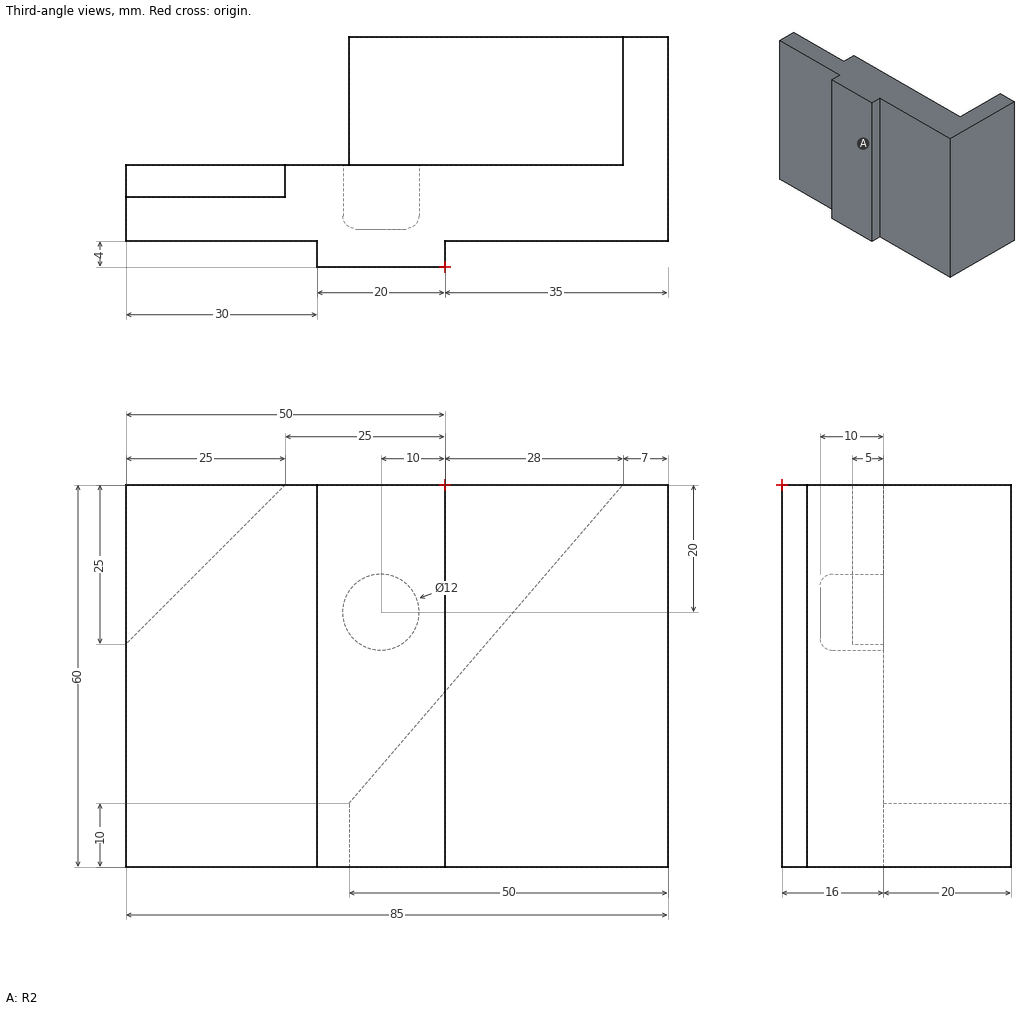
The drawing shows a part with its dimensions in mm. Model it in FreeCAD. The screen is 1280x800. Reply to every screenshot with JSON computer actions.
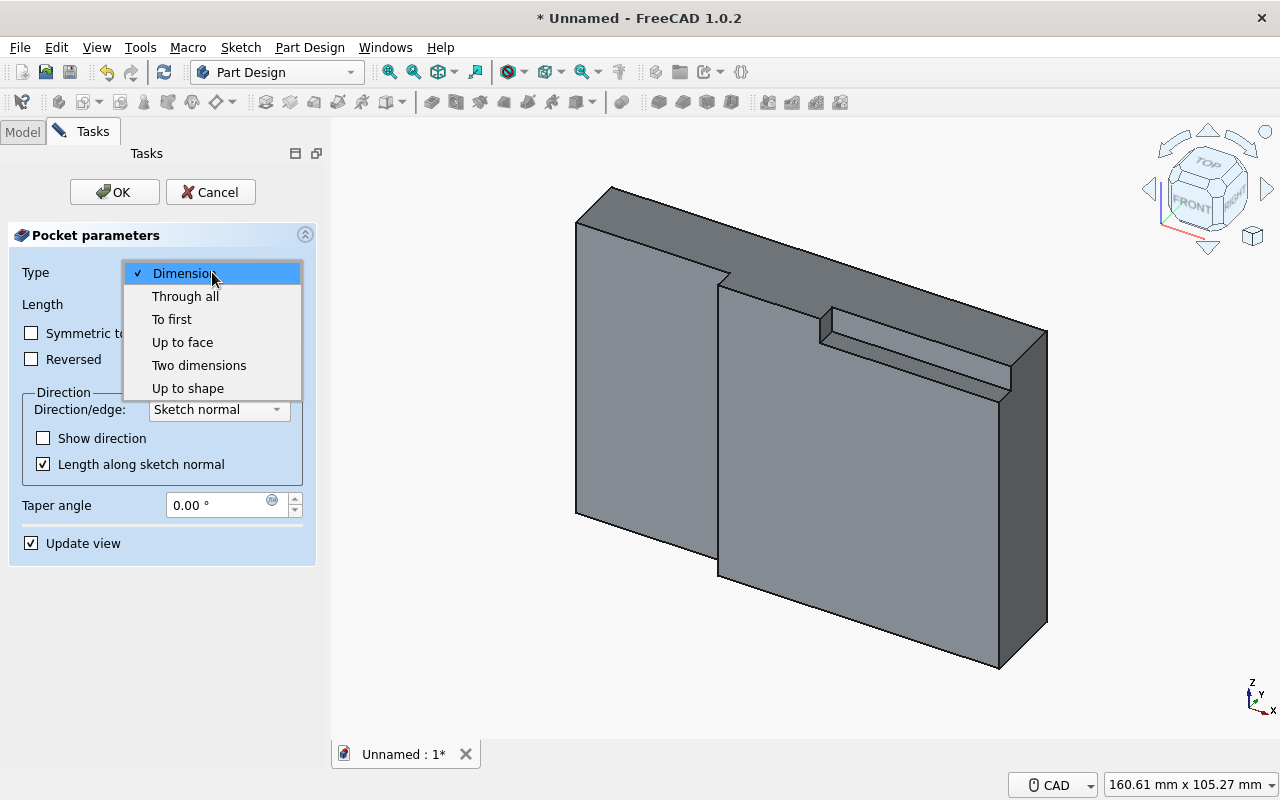
{"action": "left_click", "coordinate": [212, 296]}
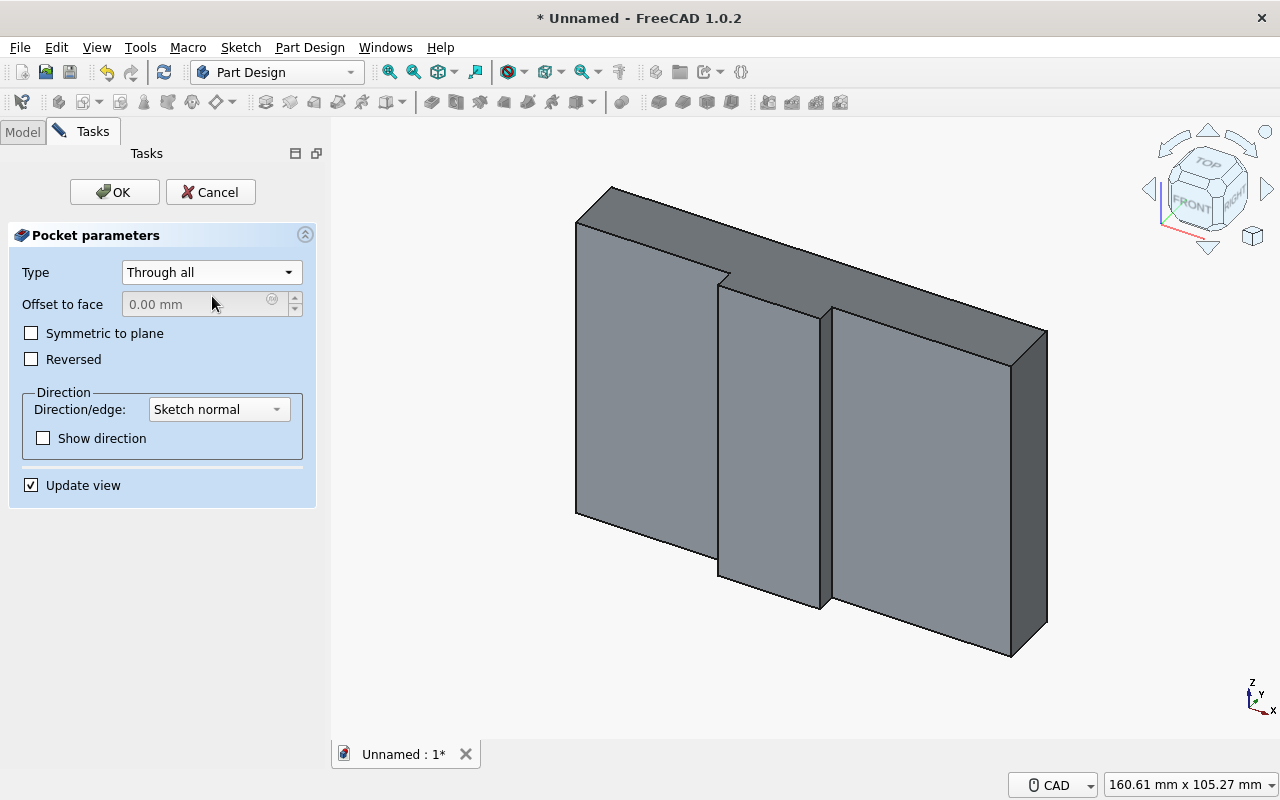
{"action": "left_click", "coordinate": [115, 192]}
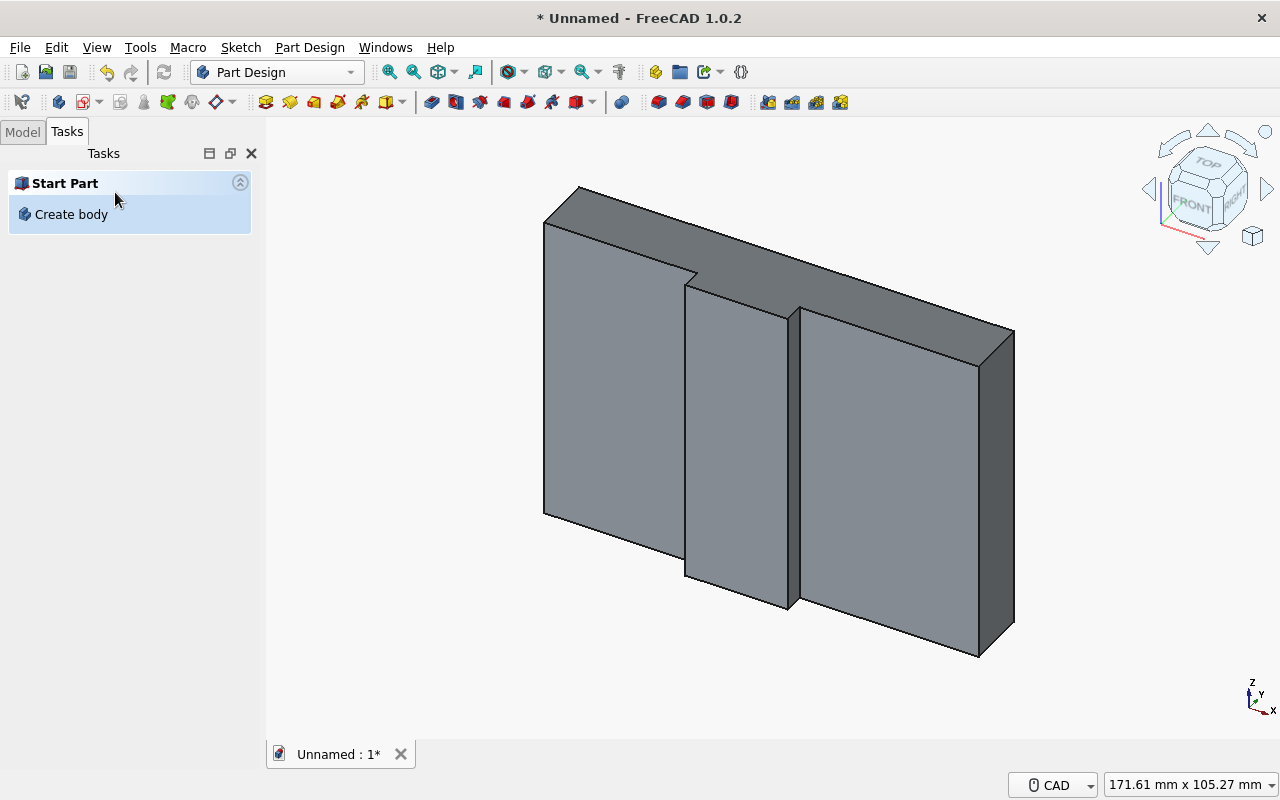
{"action": "key", "text": "4"}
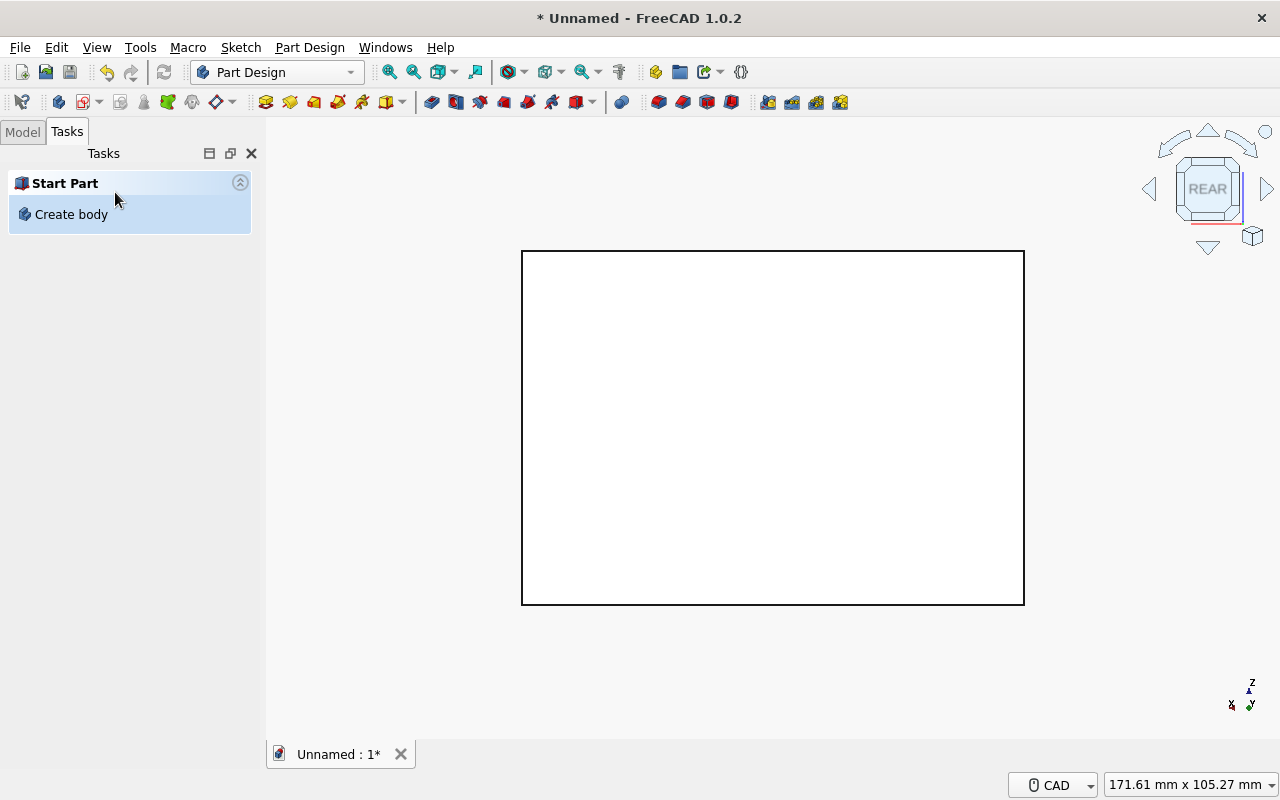
{"action": "left_click", "coordinate": [701, 427]}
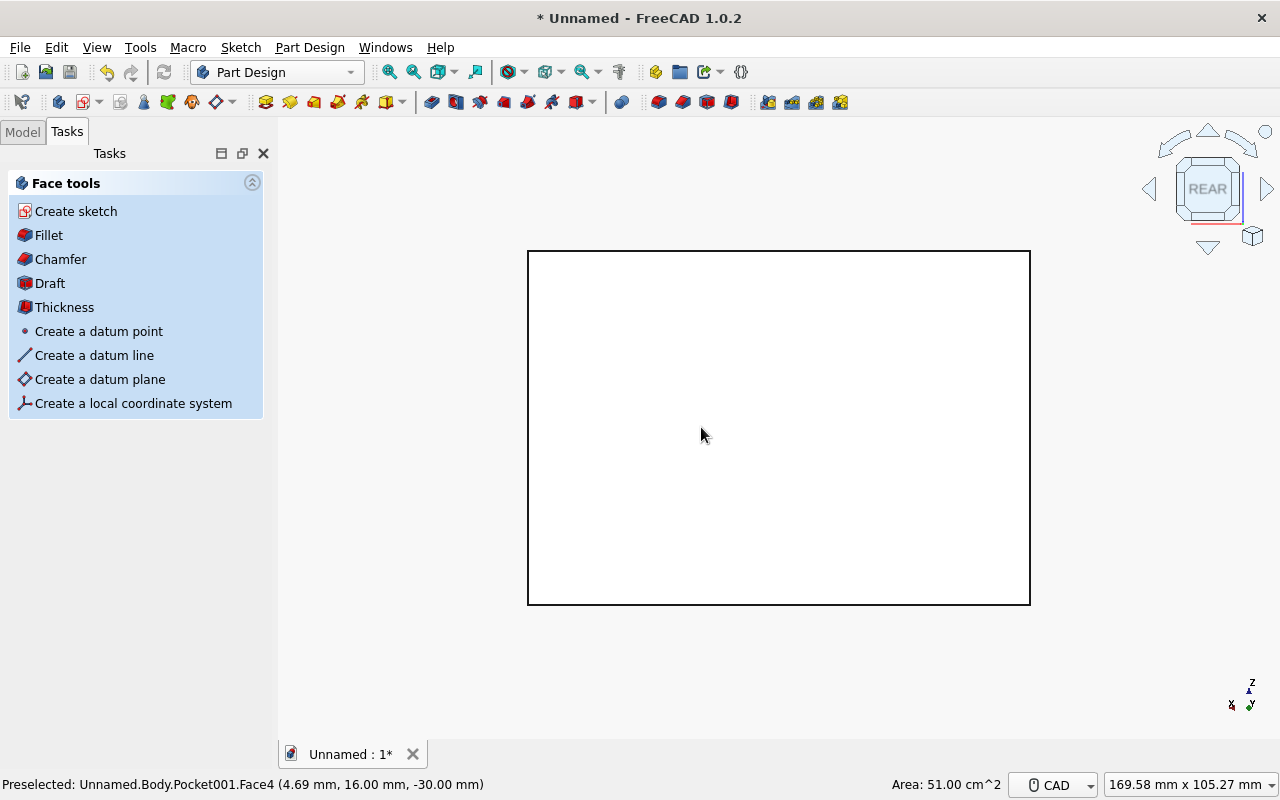
{"action": "left_click", "coordinate": [84, 102]}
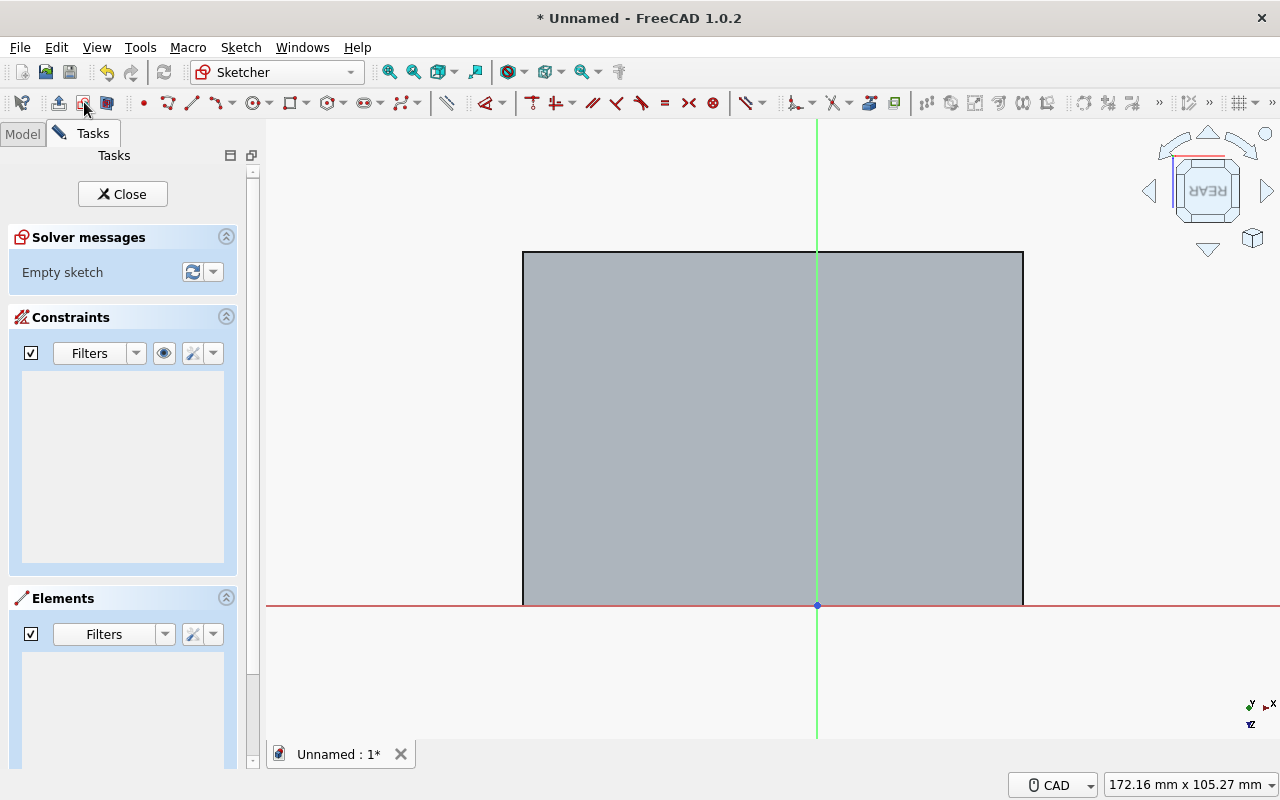
{"action": "left_click", "coordinate": [168, 104]}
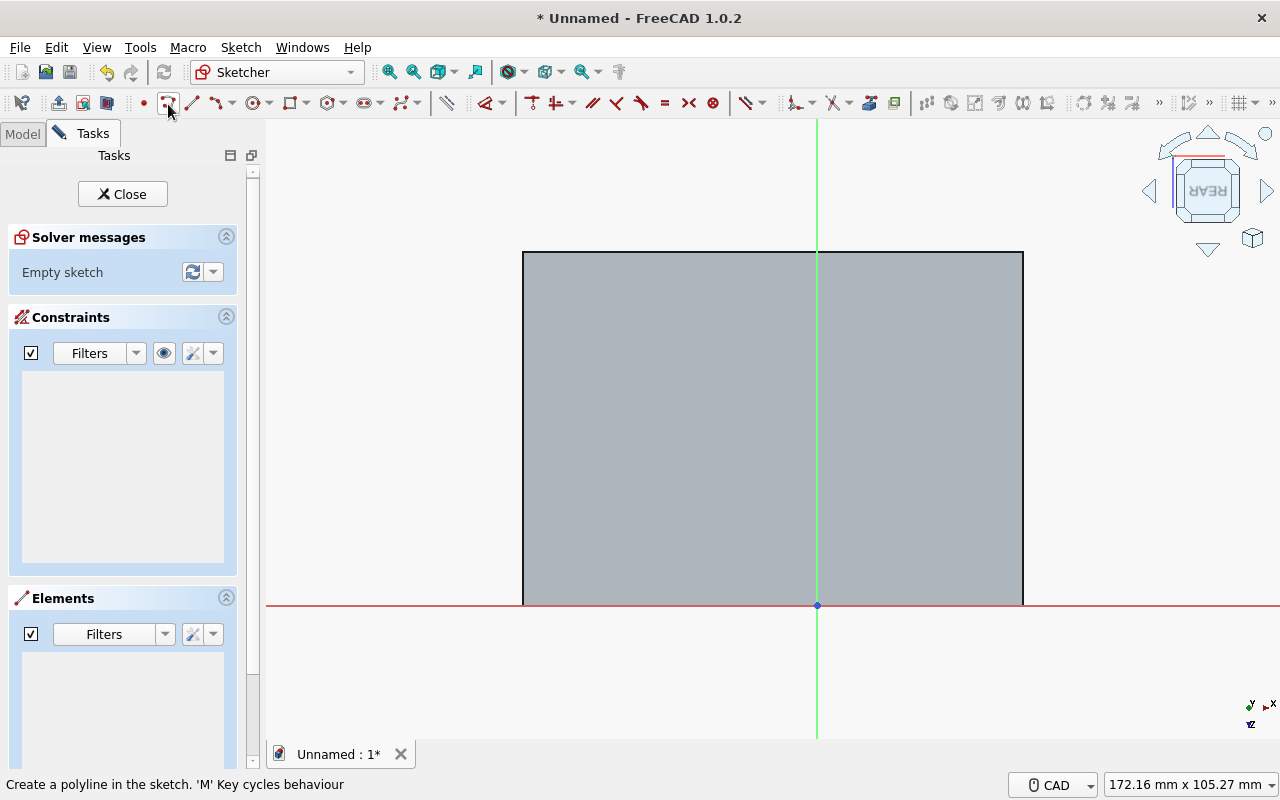
{"action": "left_click", "coordinate": [982, 606]}
{"action": "left_click", "coordinate": [1023, 597]}
{"action": "left_click", "coordinate": [1023, 252]}
{"action": "left_click", "coordinate": [729, 252]}
{"action": "left_click", "coordinate": [729, 311]}
{"action": "left_click", "coordinate": [982, 606]}
{"action": "key", "text": "Escape"}
{"action": "key", "text": "Escape"}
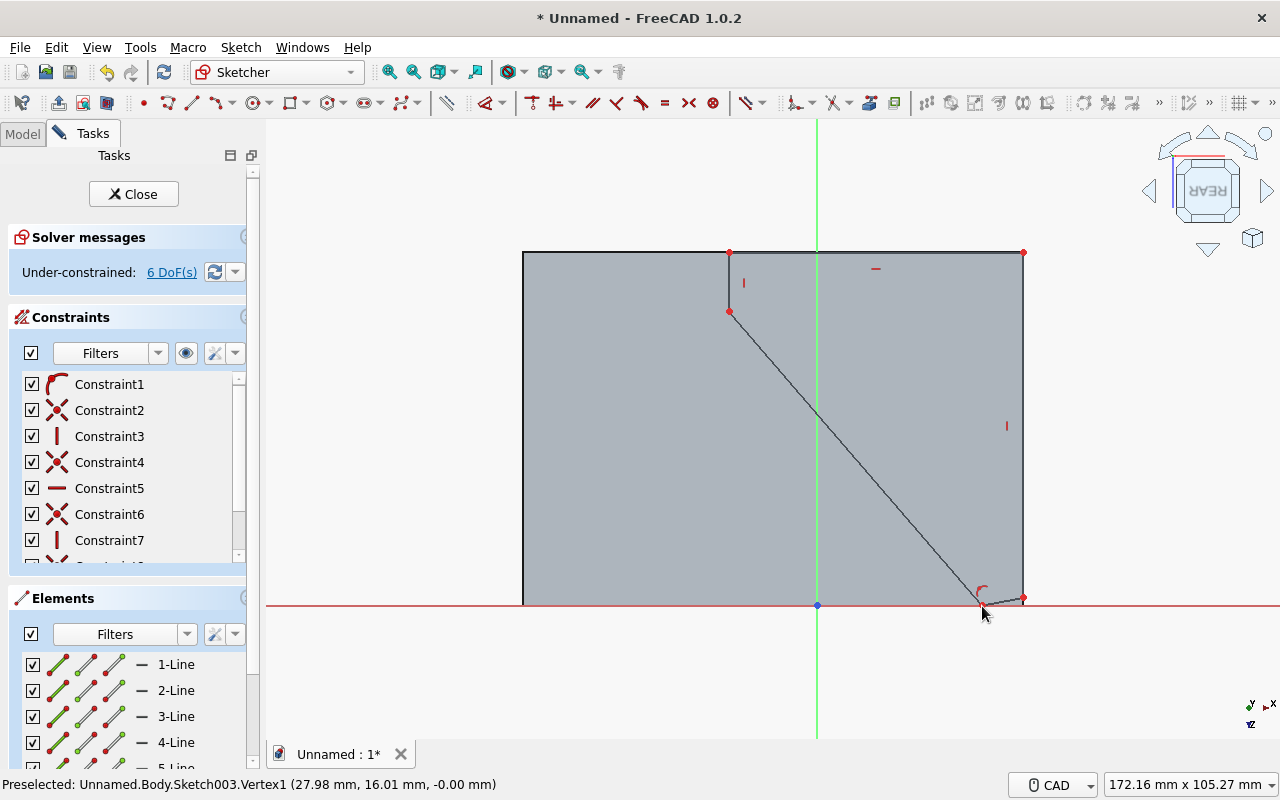
{"action": "left_click", "coordinate": [994, 603]}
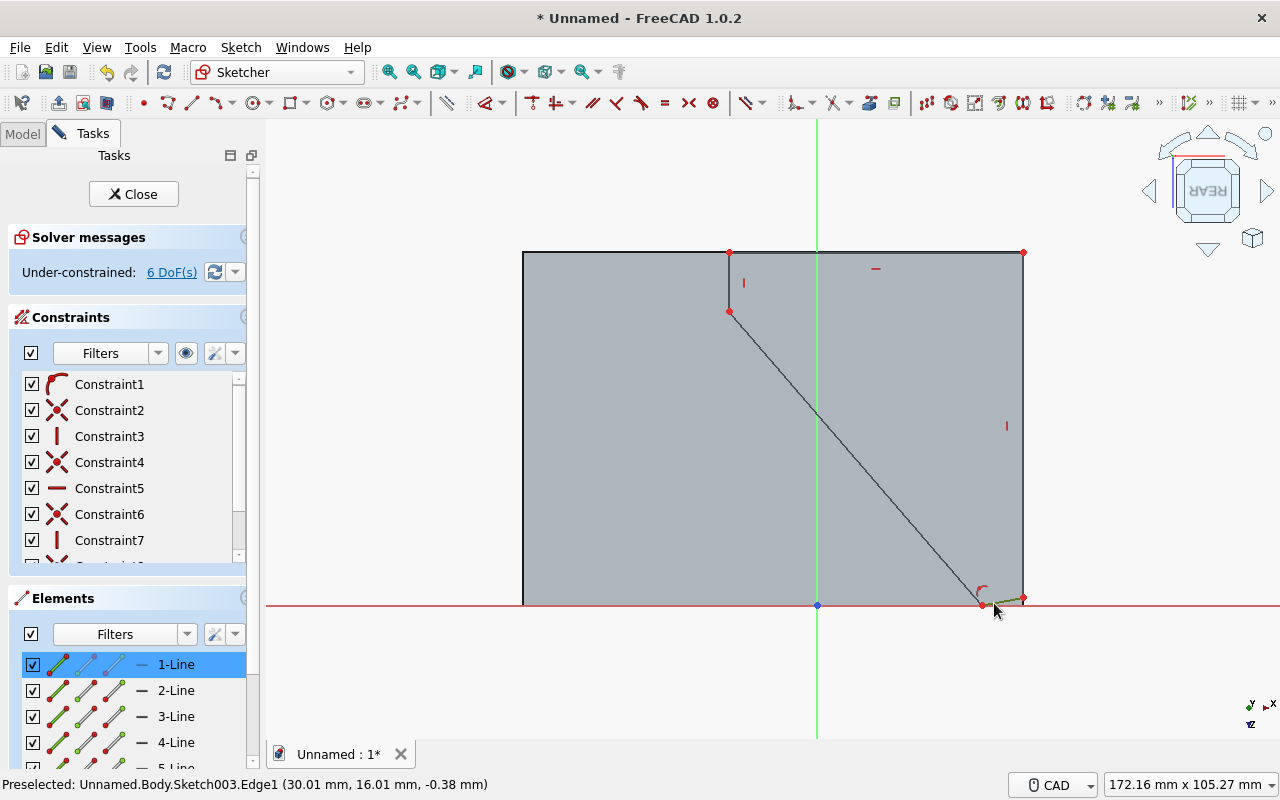
{"action": "key", "text": "h"}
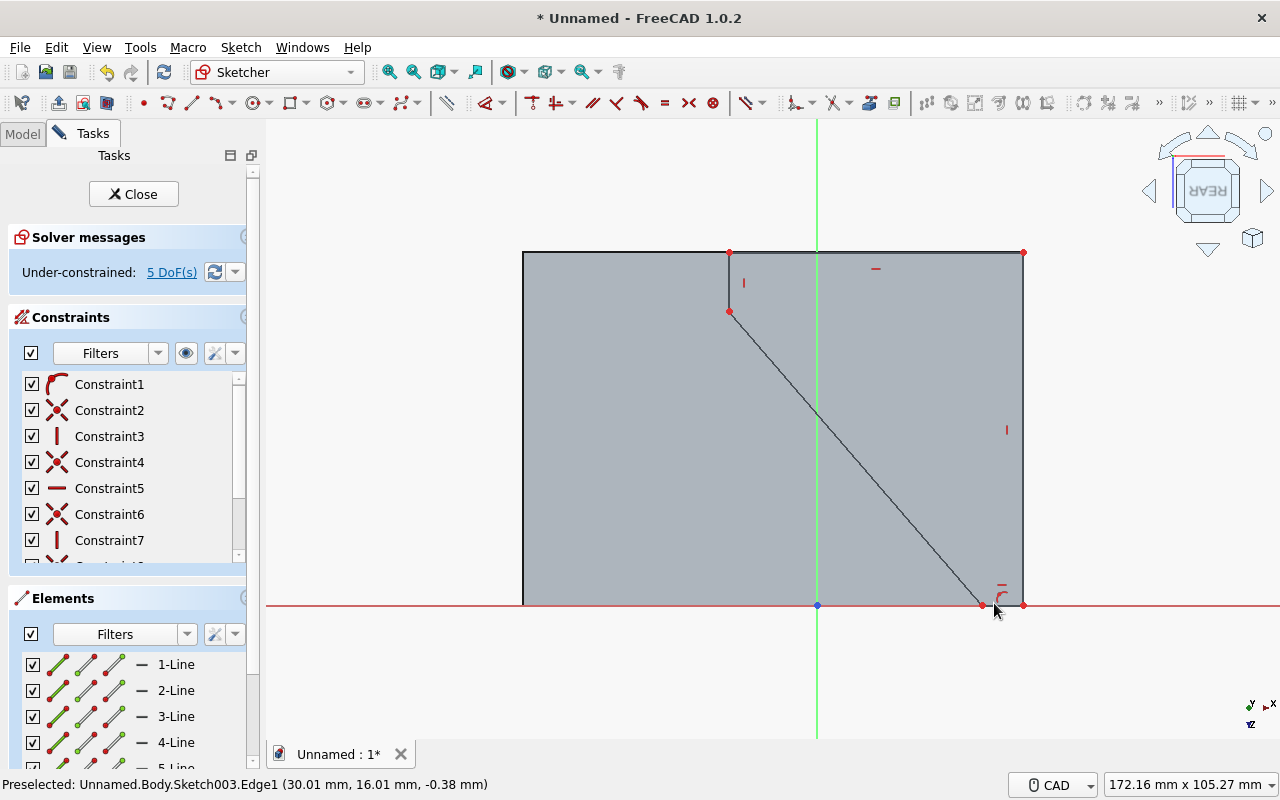
{"action": "left_click", "coordinate": [486, 104]}